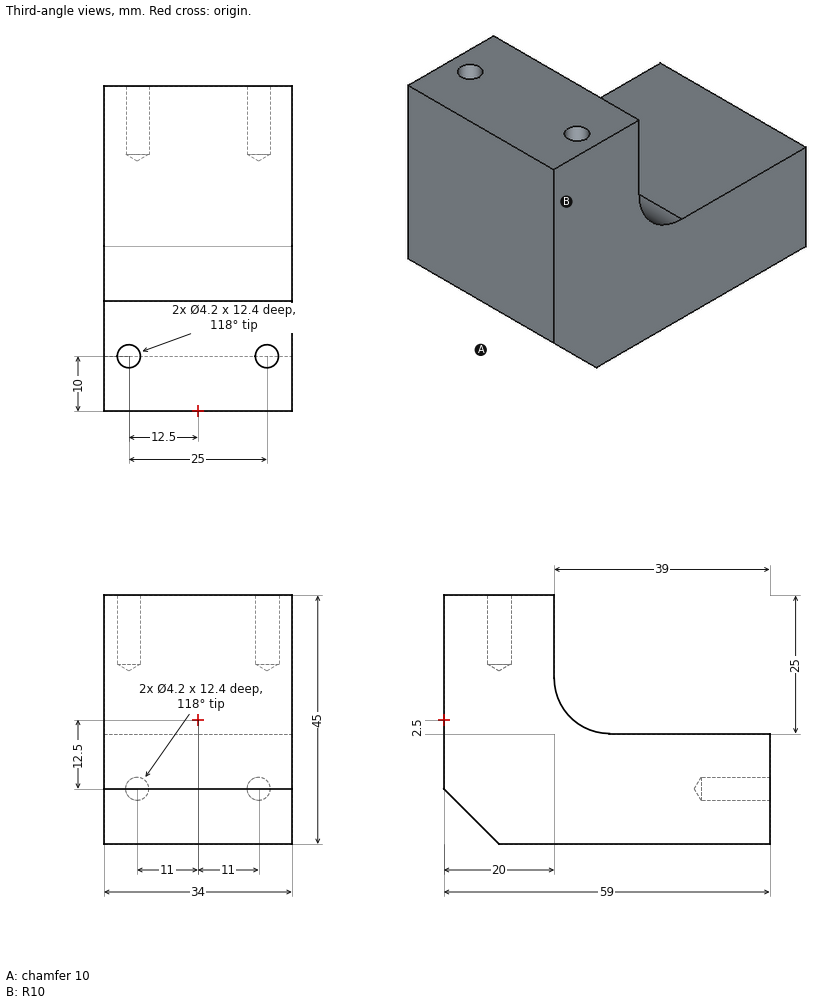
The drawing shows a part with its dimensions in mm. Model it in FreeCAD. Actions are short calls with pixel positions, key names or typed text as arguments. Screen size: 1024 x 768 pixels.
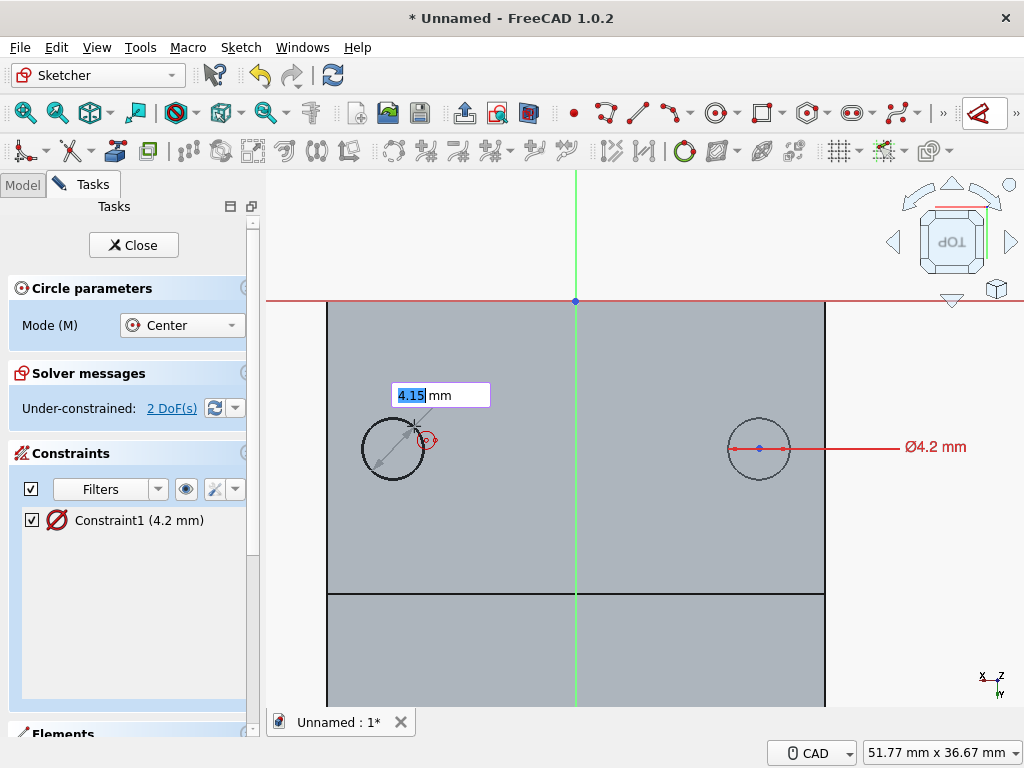
text(4.2)
key(Return)
key(Escape)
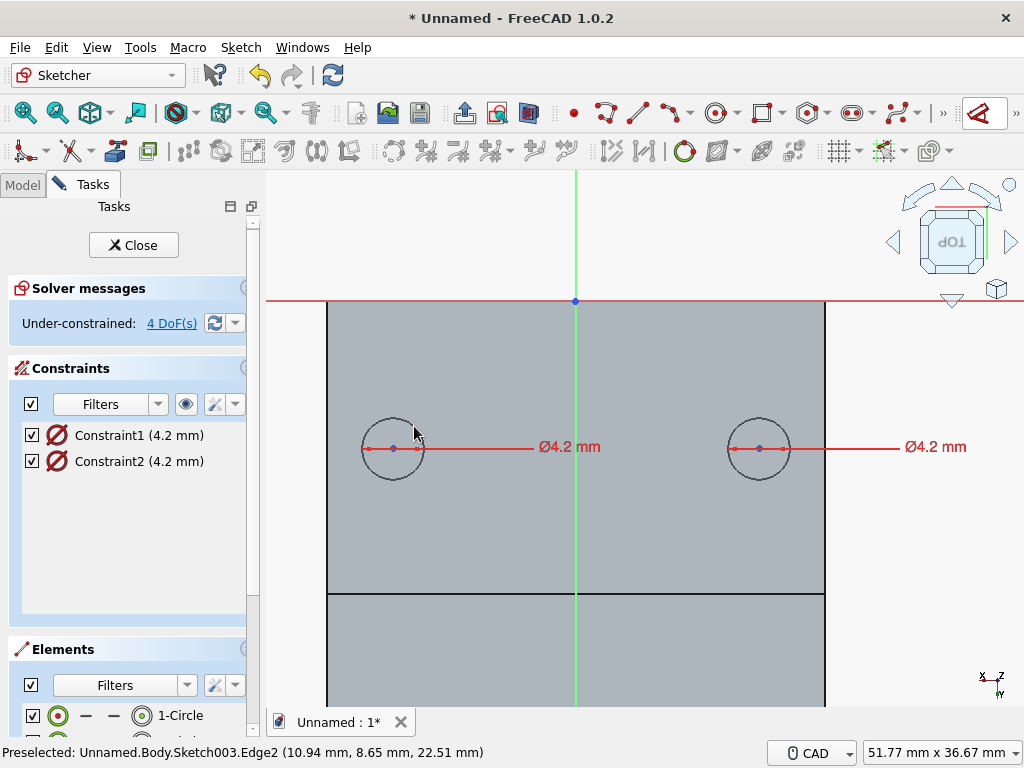
click(759, 449)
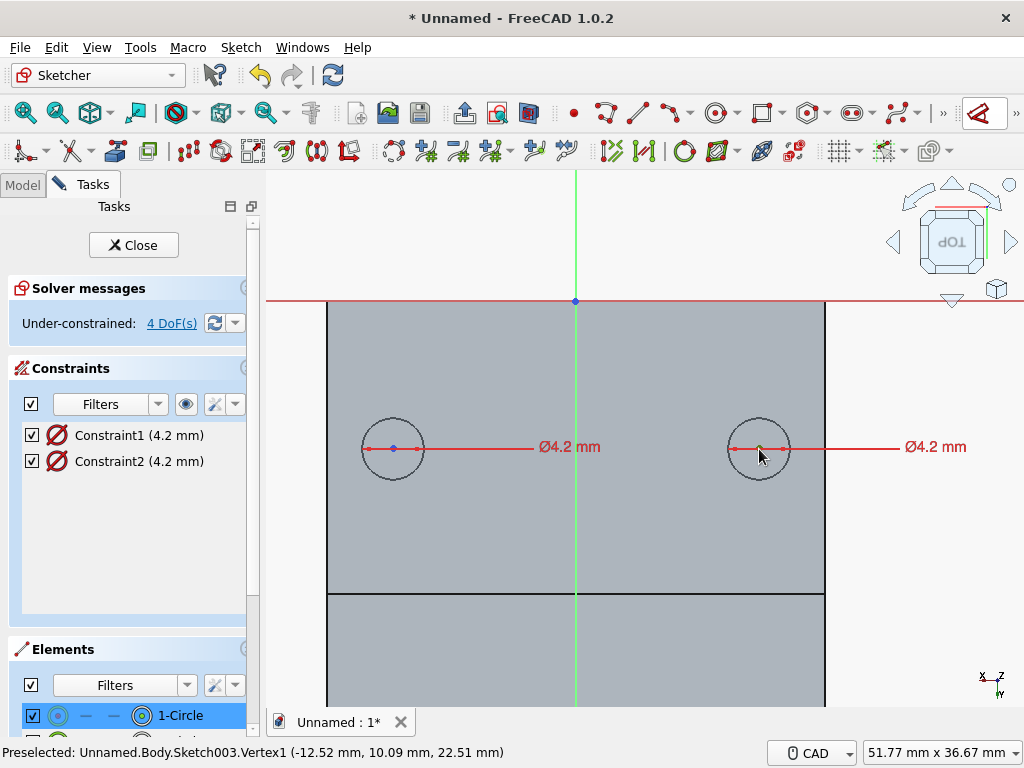
click(393, 449)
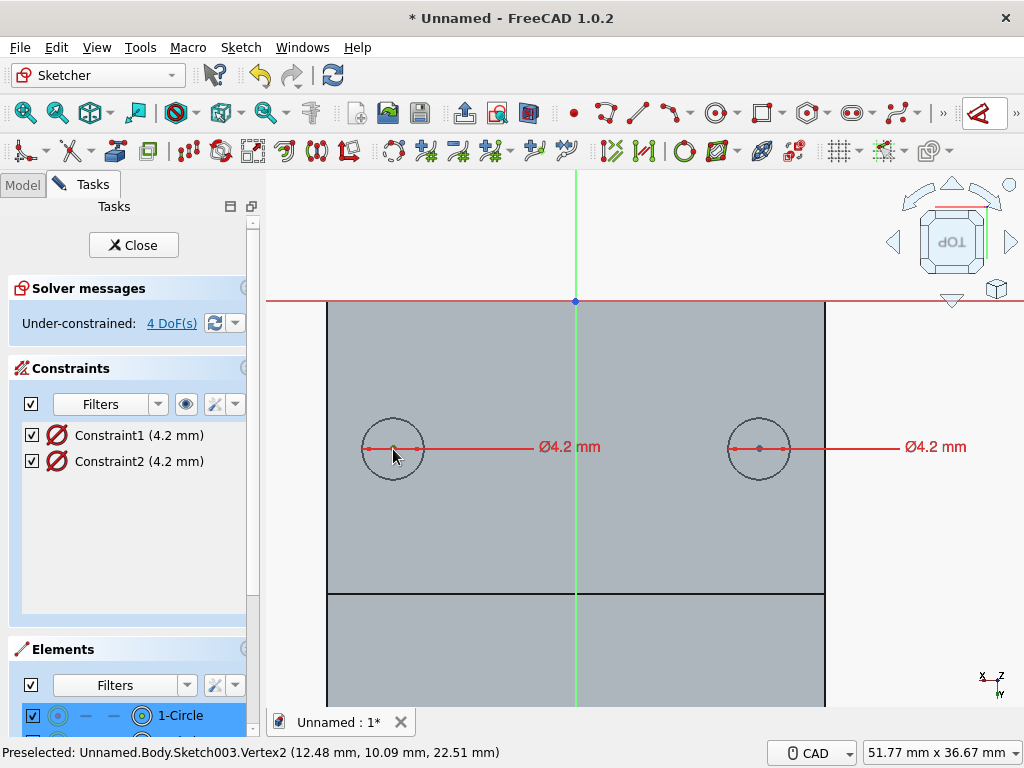
key(h)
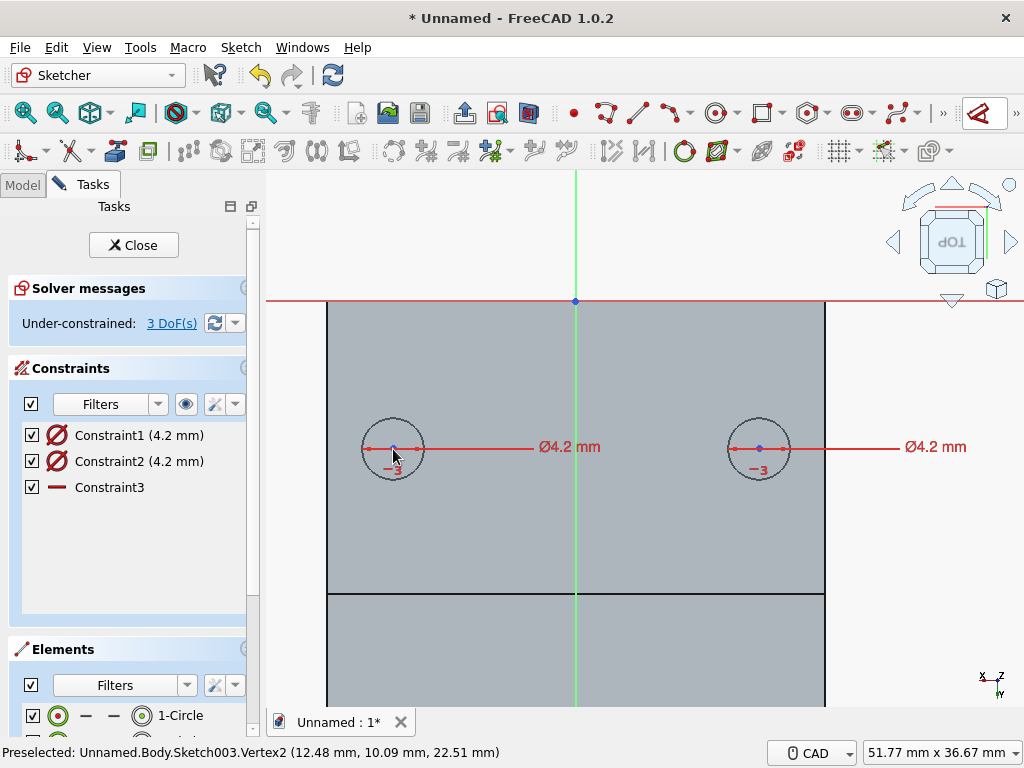
click(759, 449)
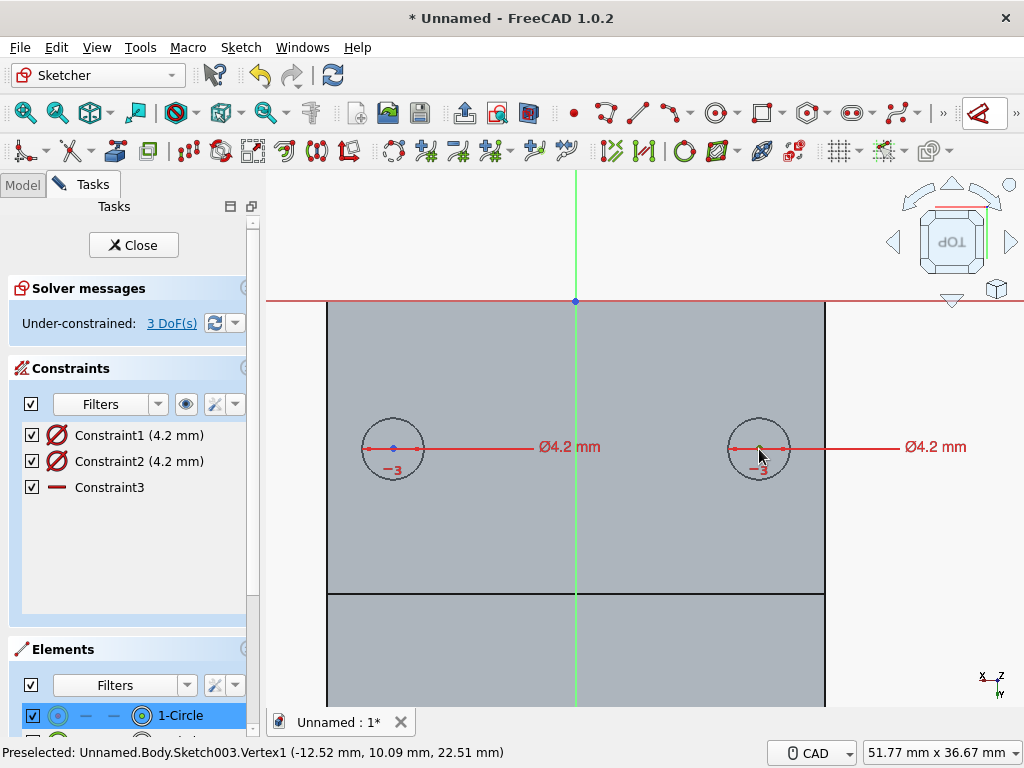
click(1002, 114)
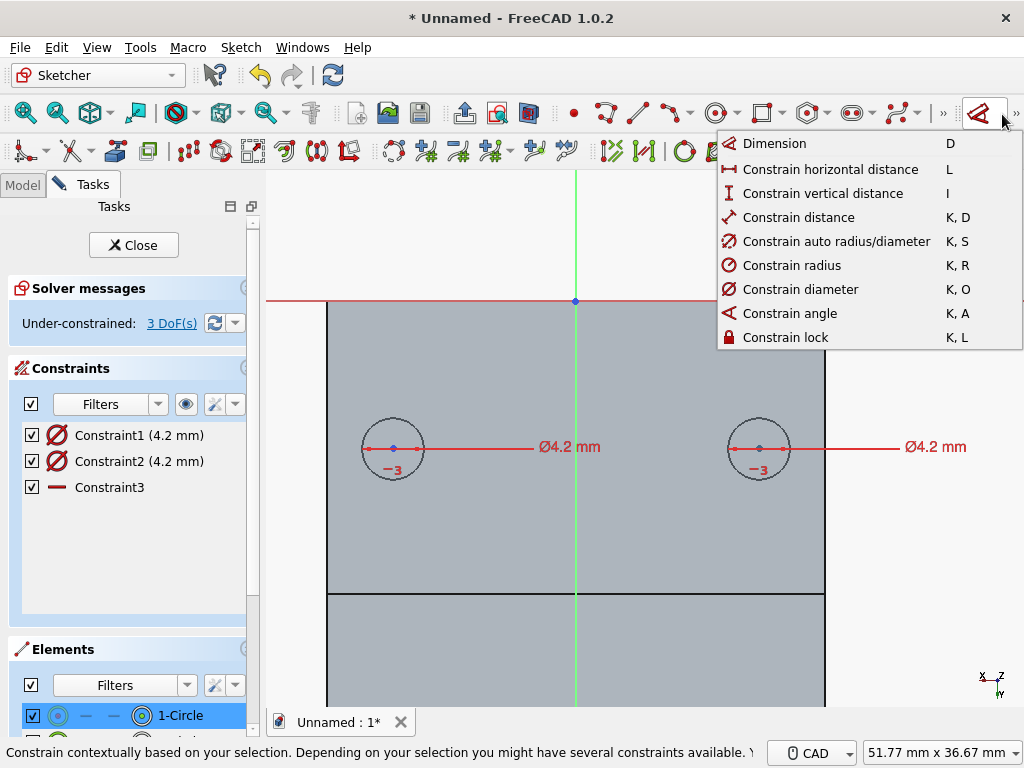
click(870, 193)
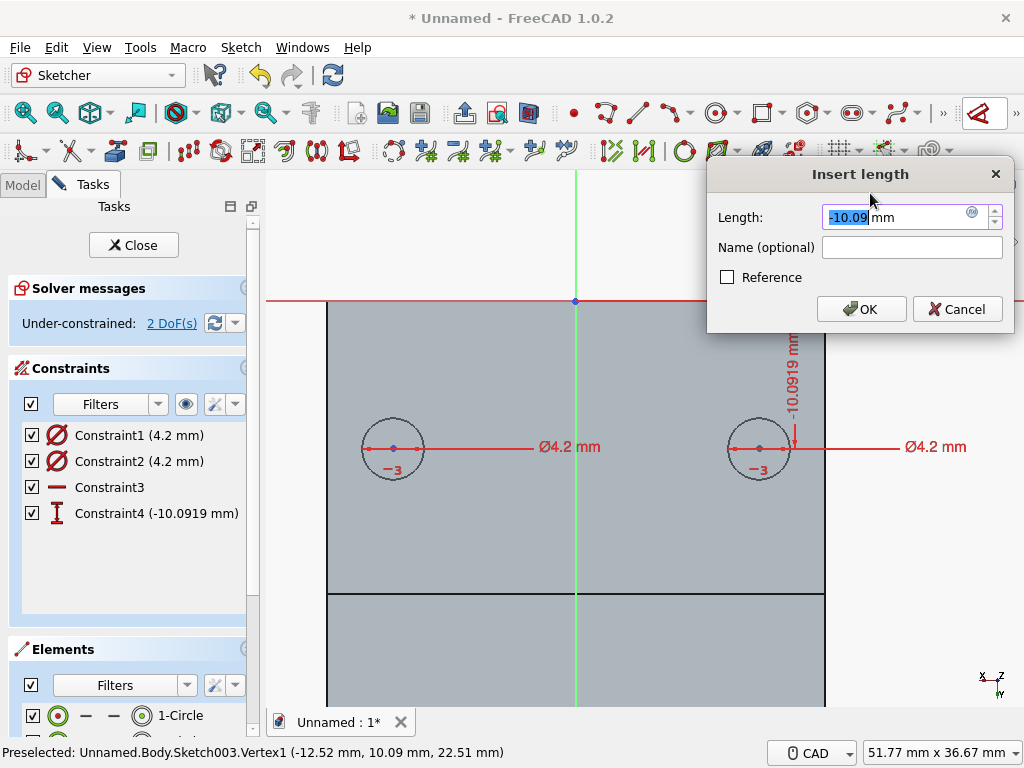
text(-10)
key(Return)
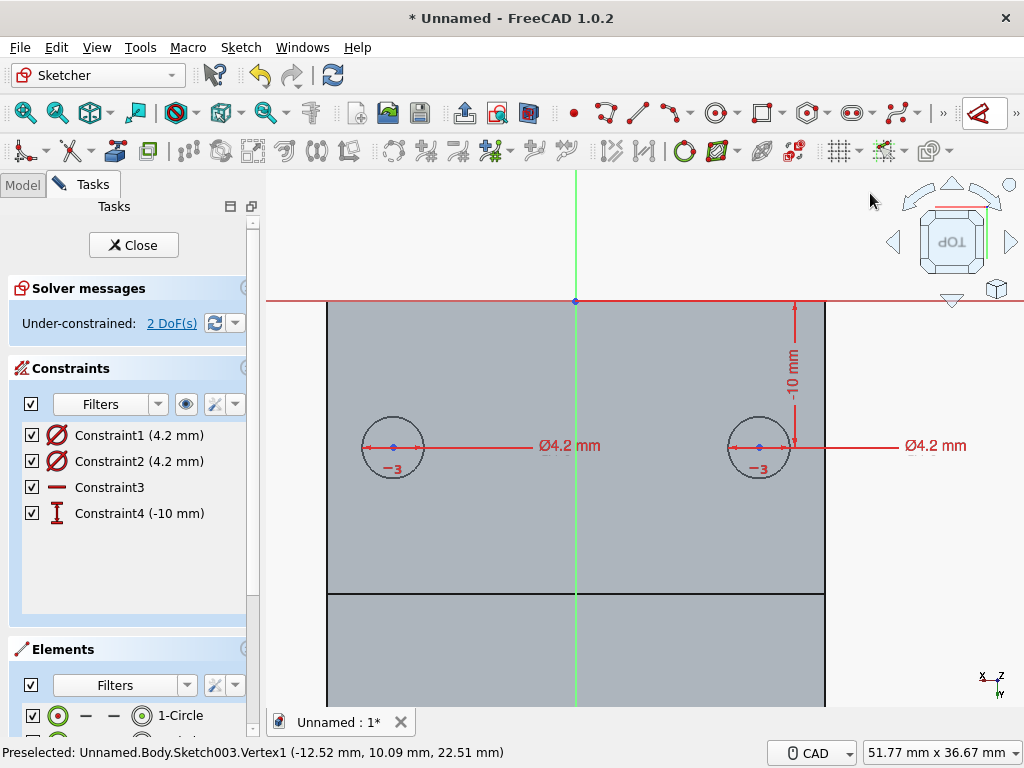
click(759, 448)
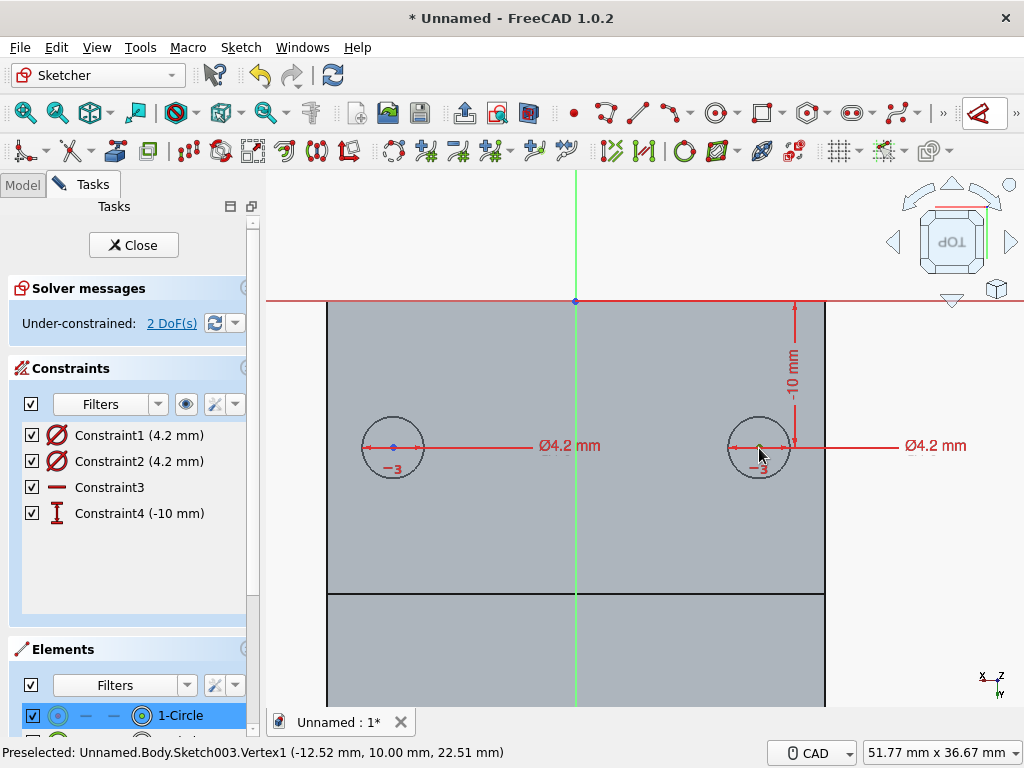
click(393, 448)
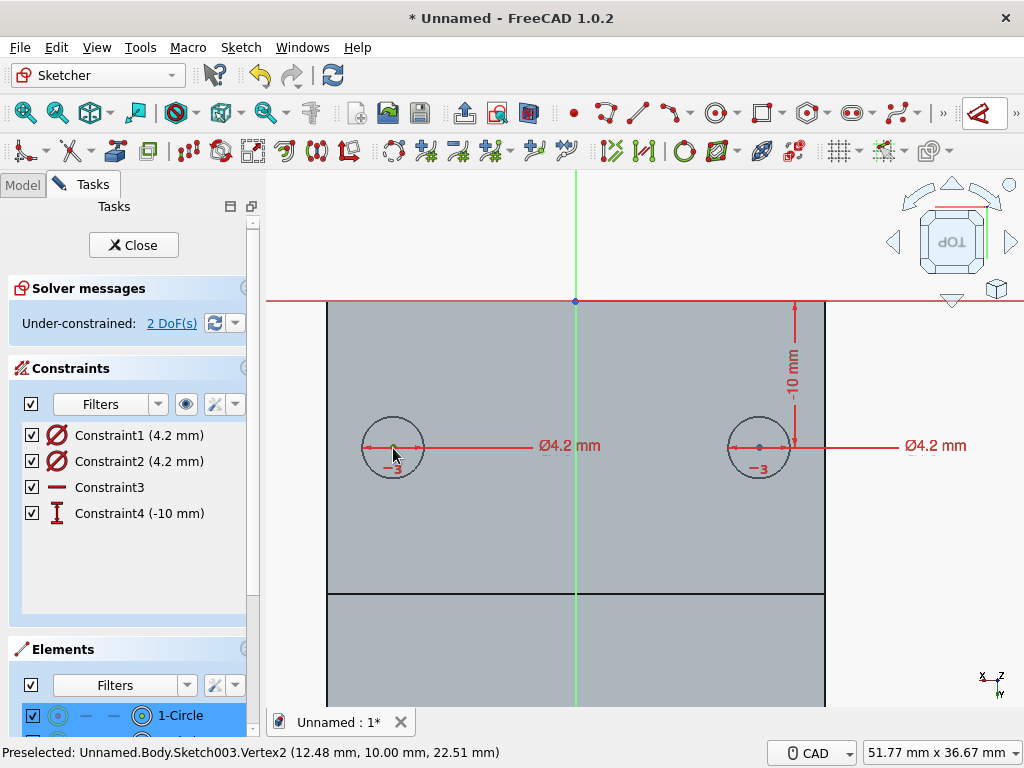
key(l)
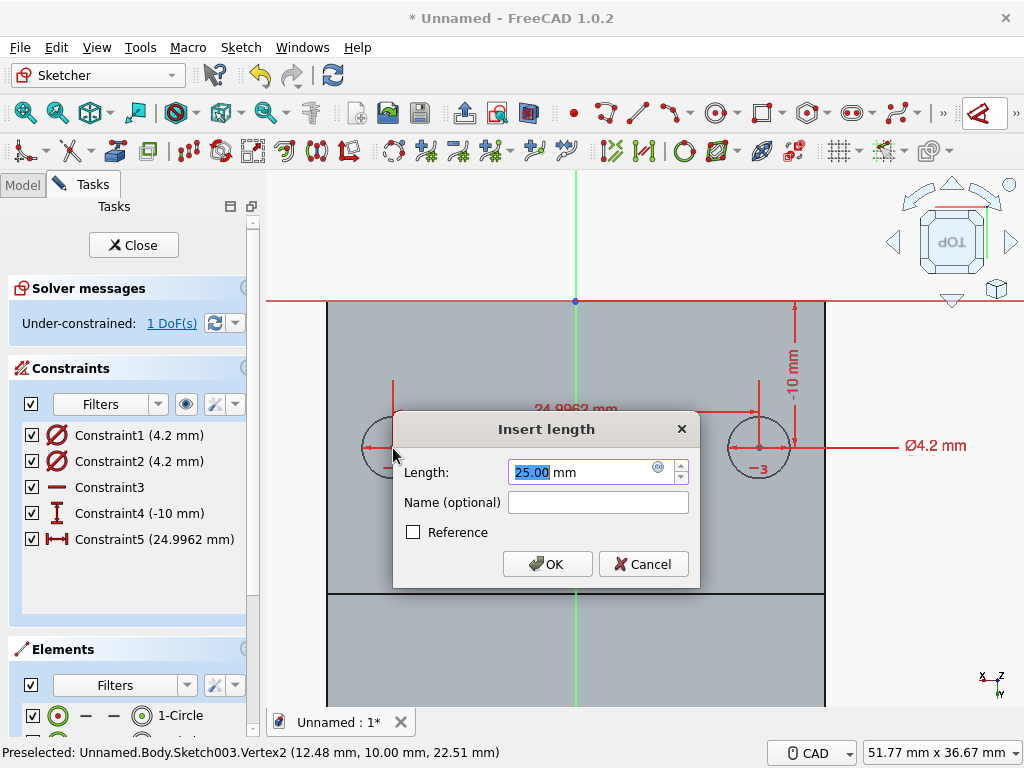
text(25)
key(Return)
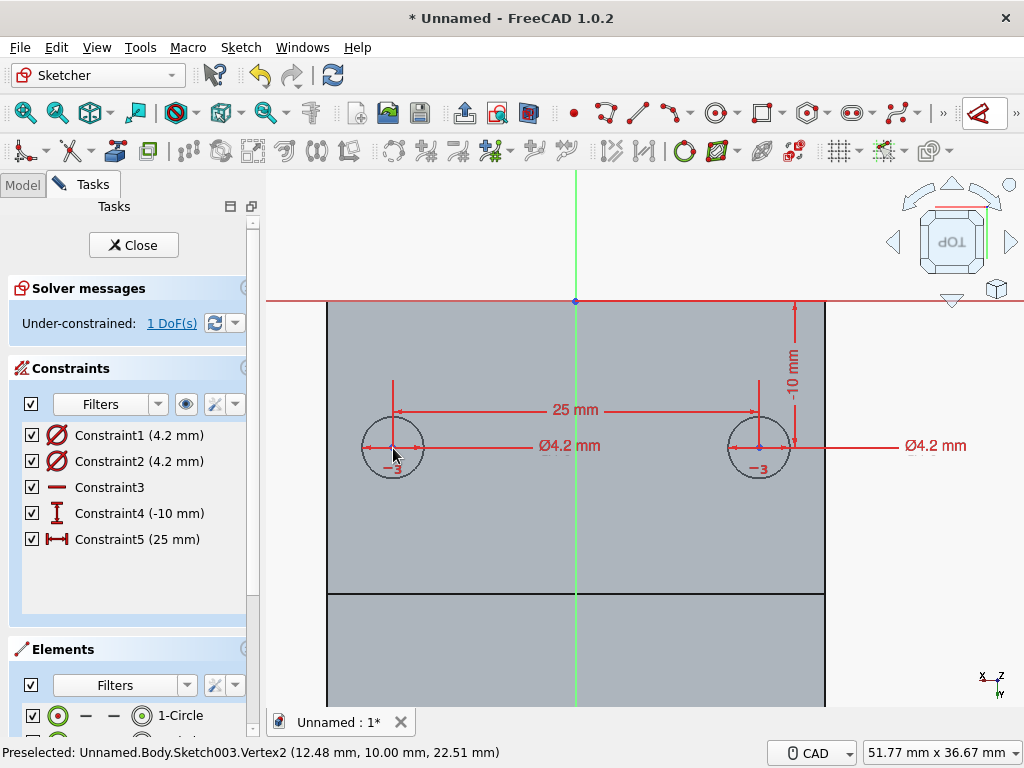
click(759, 448)